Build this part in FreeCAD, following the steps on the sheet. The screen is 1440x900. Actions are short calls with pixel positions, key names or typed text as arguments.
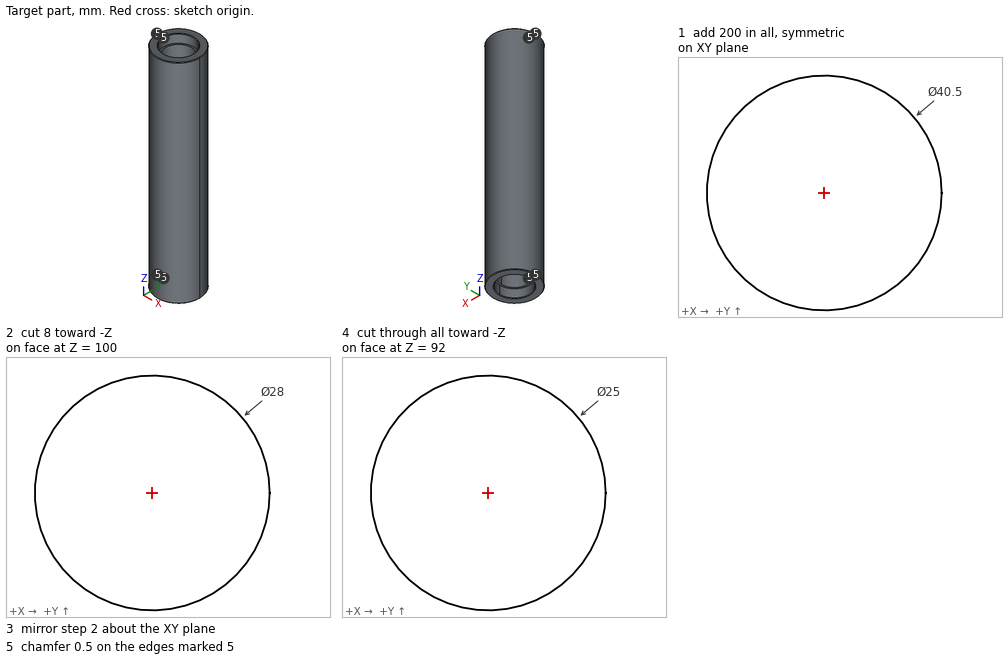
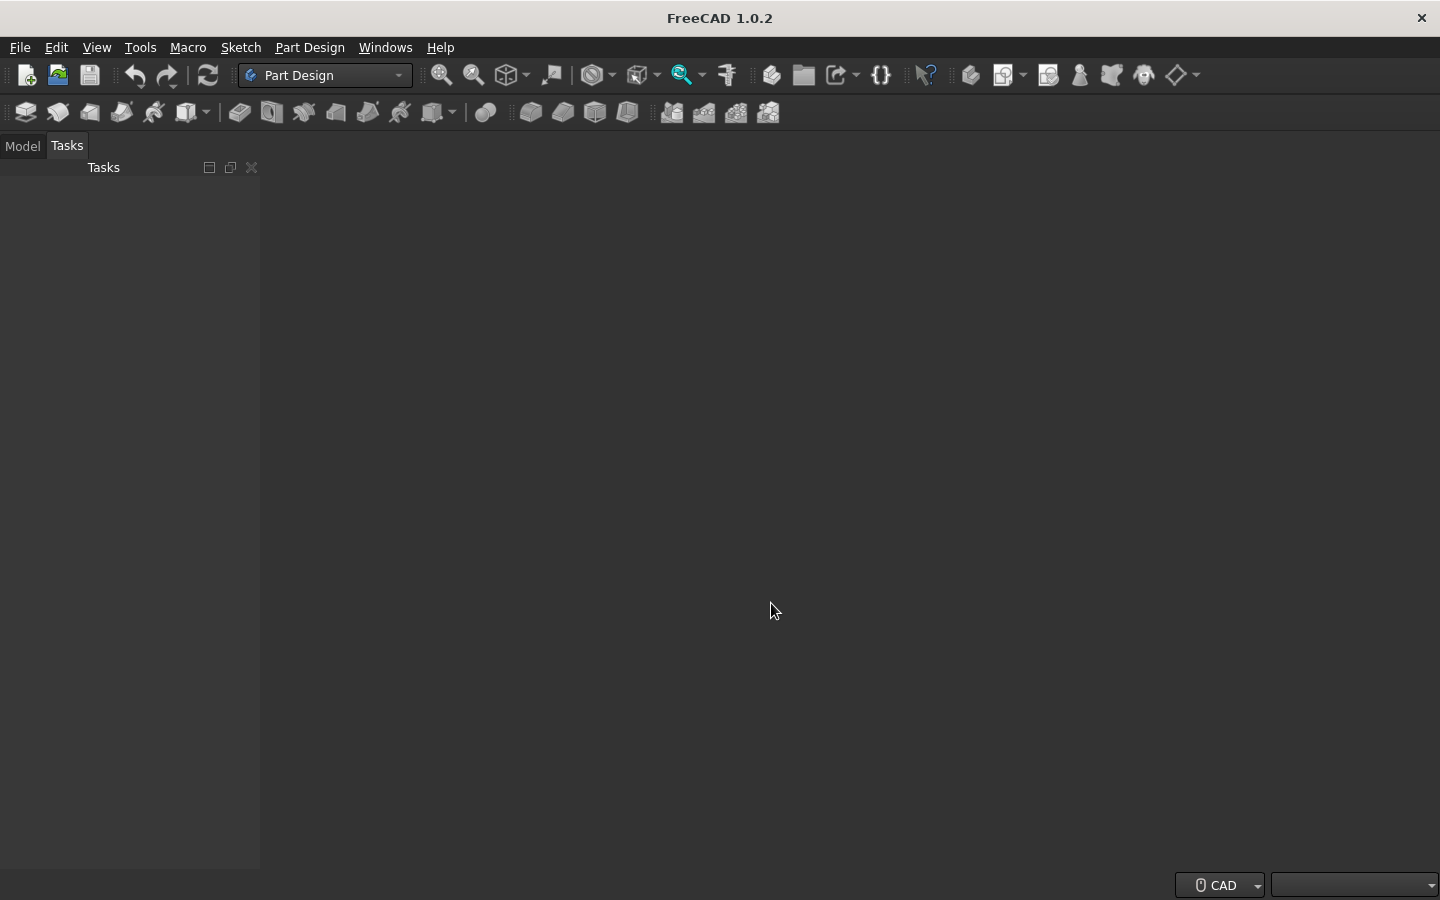
click(26, 76)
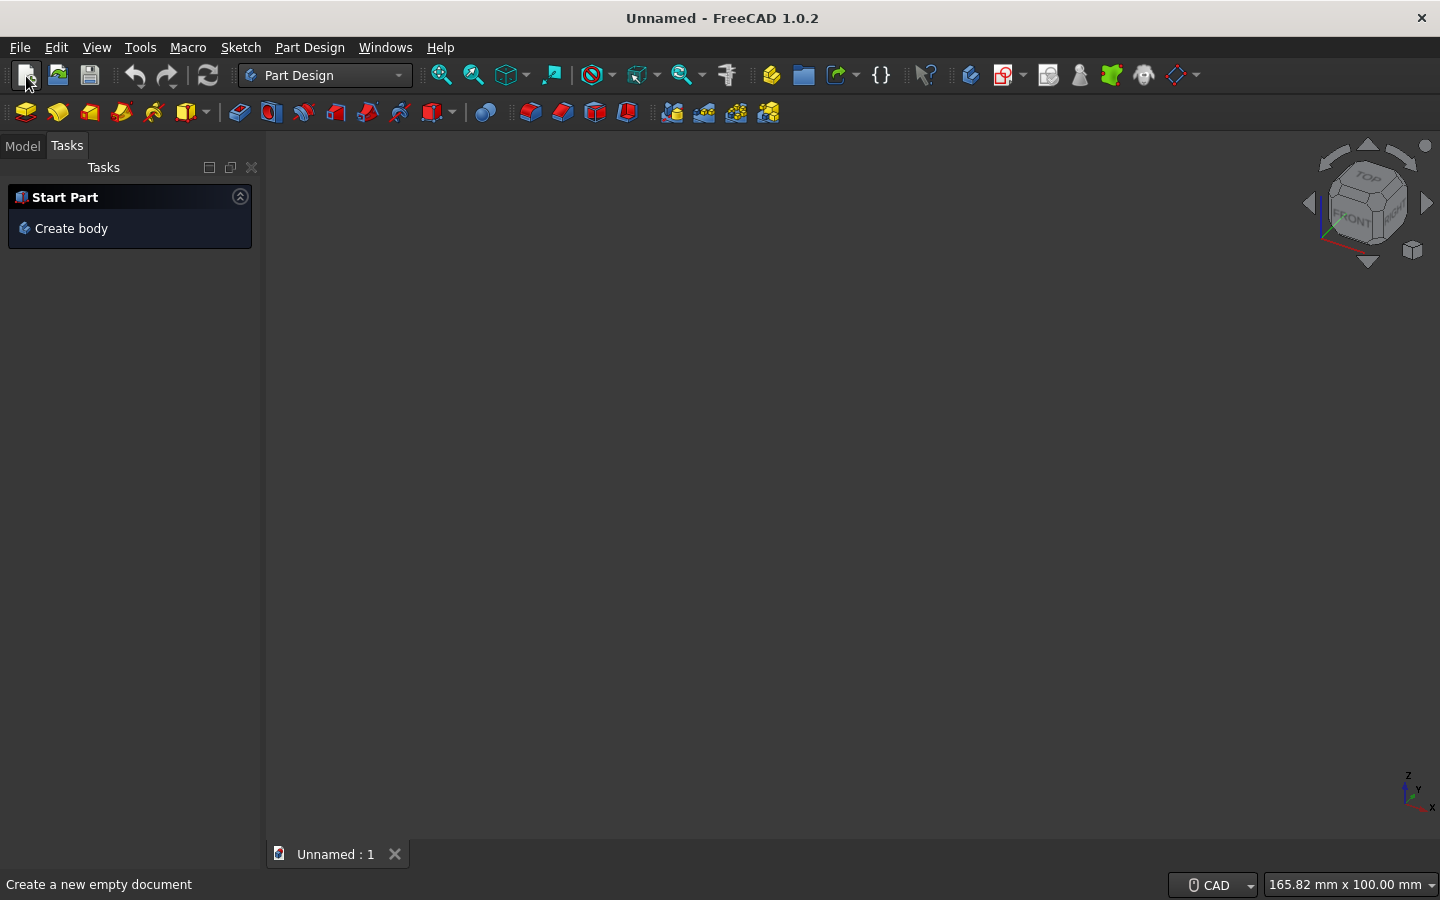
click(1004, 76)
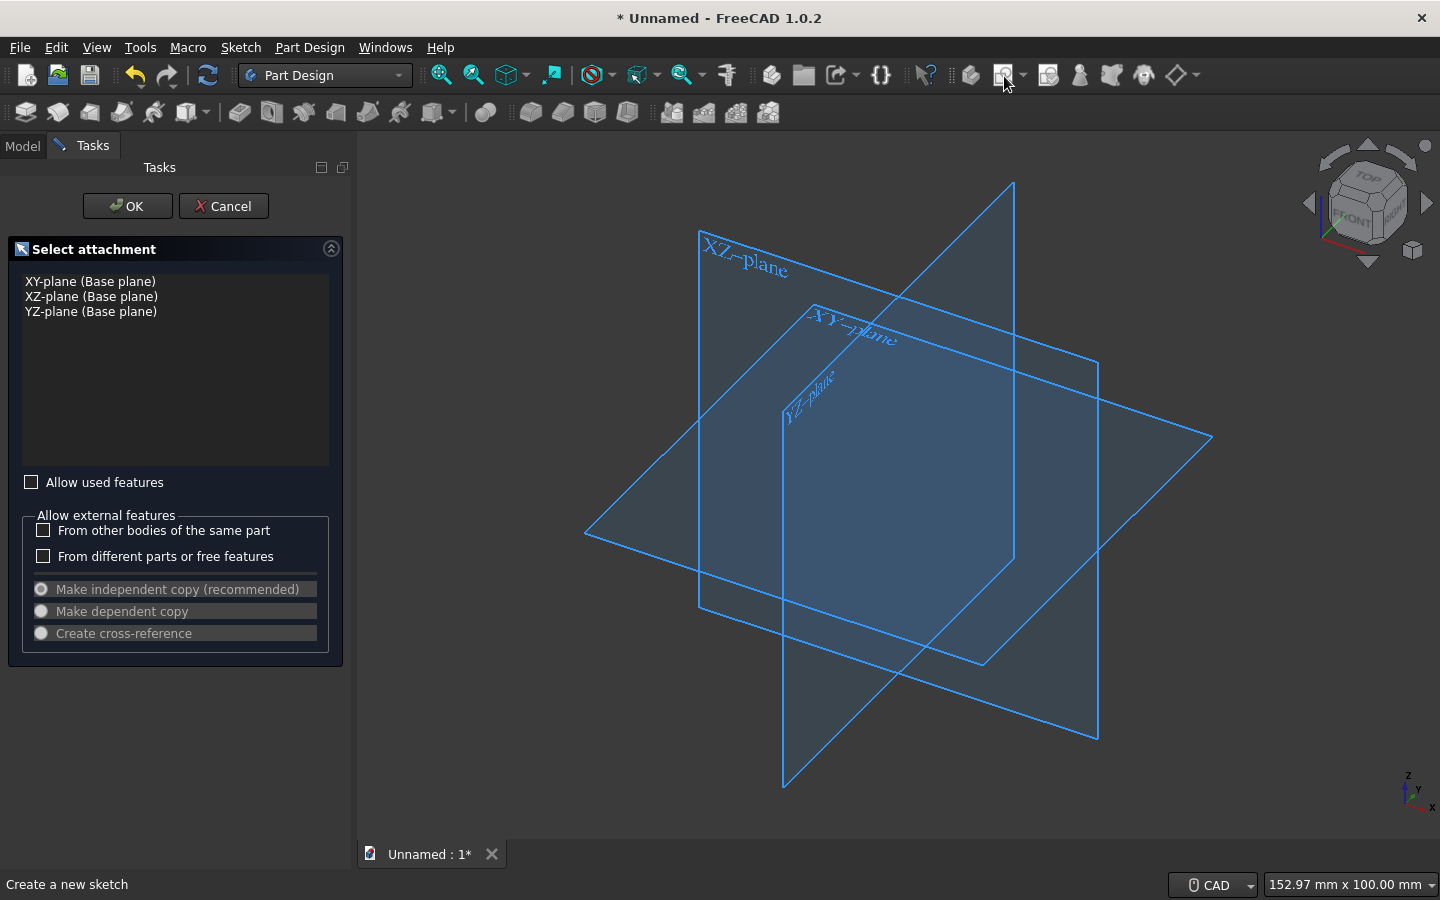
click(82, 282)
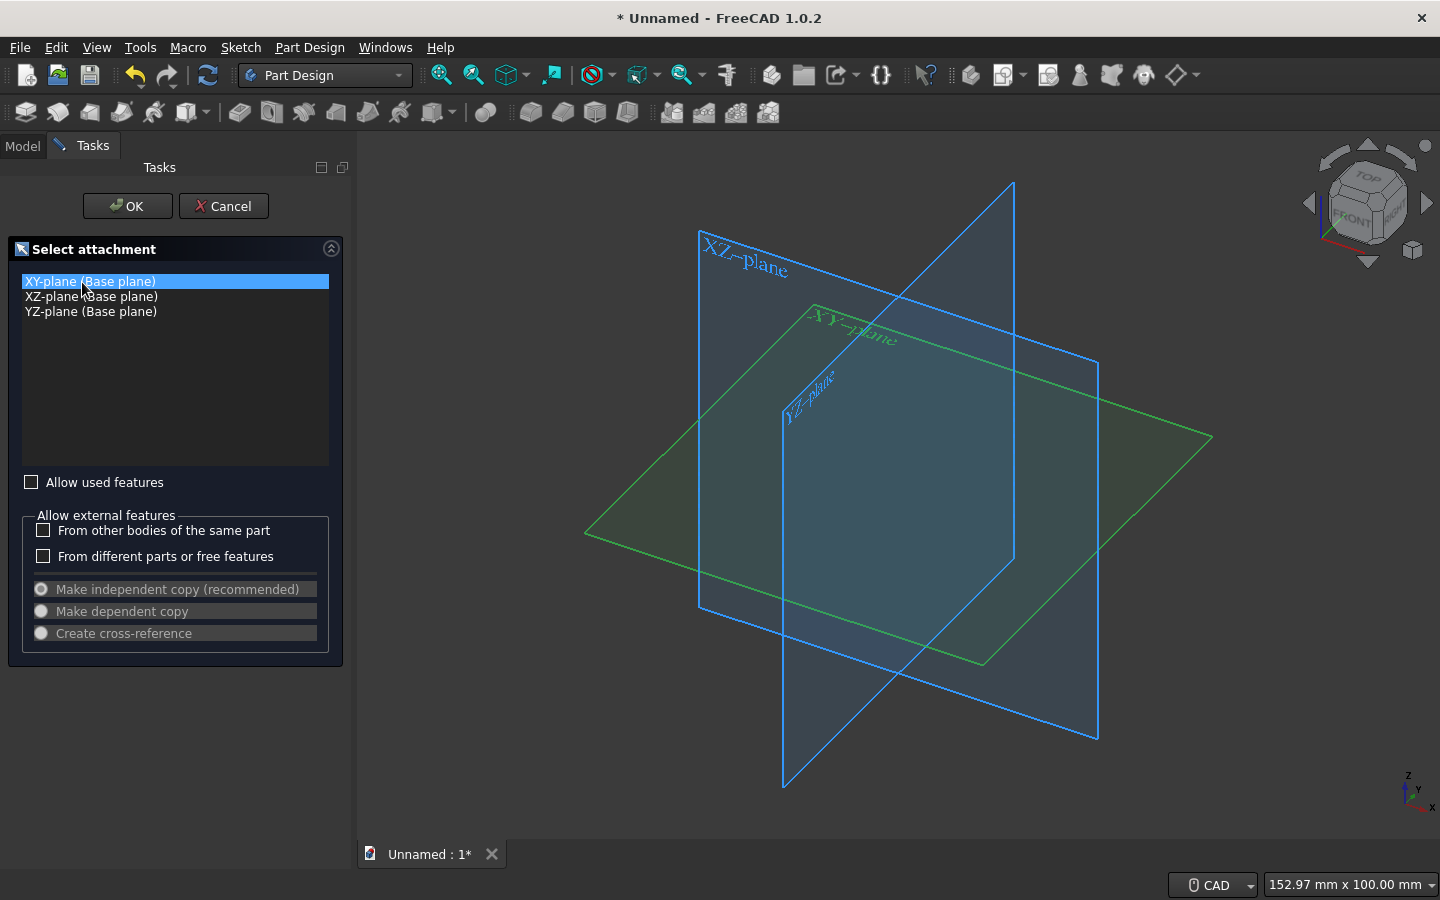
click(128, 206)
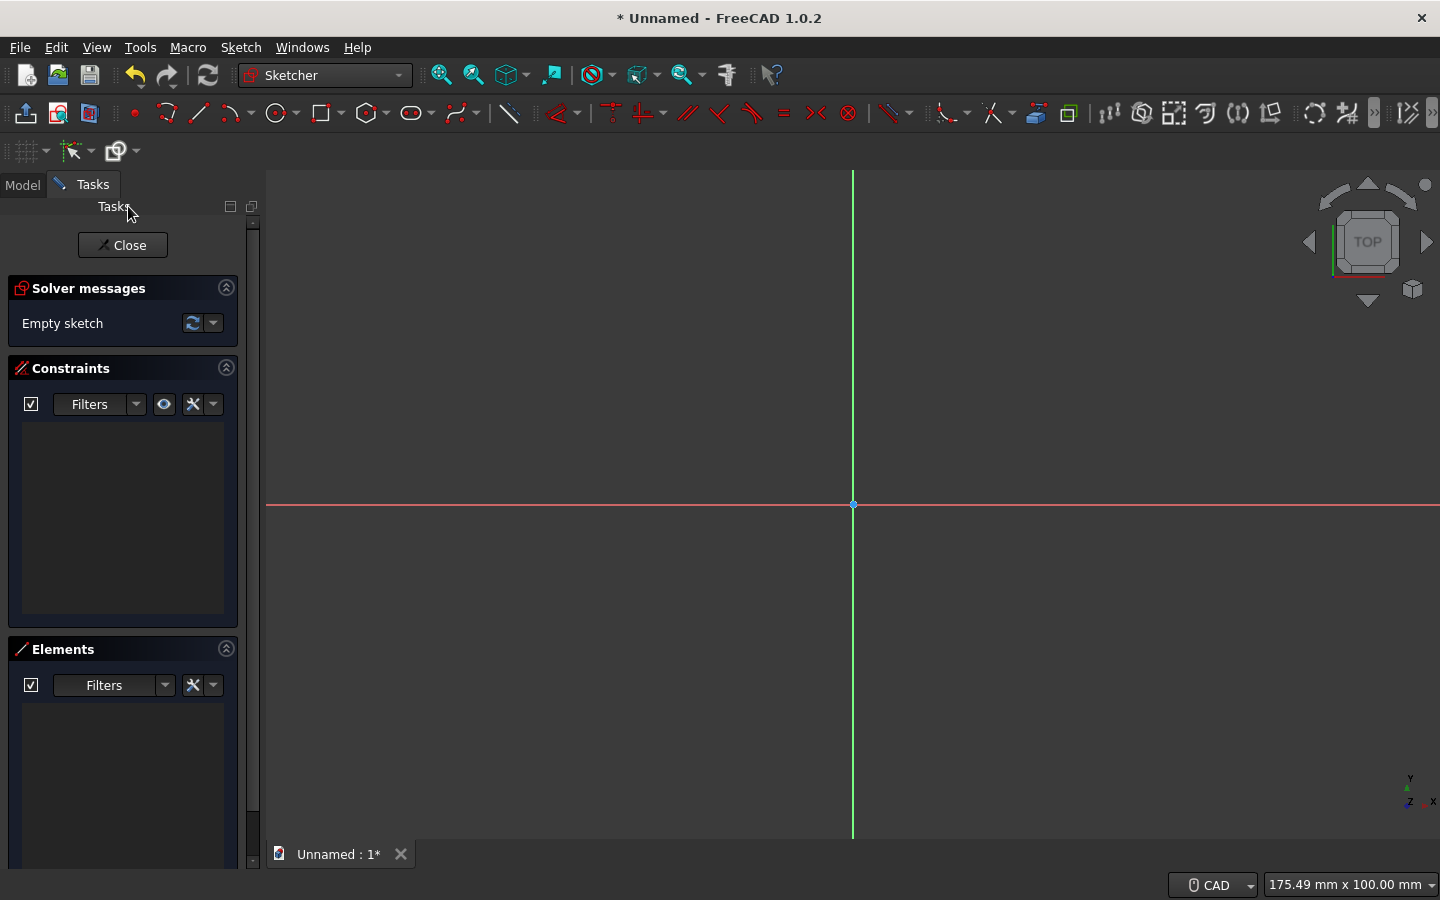
scroll(992, 504, up, 2)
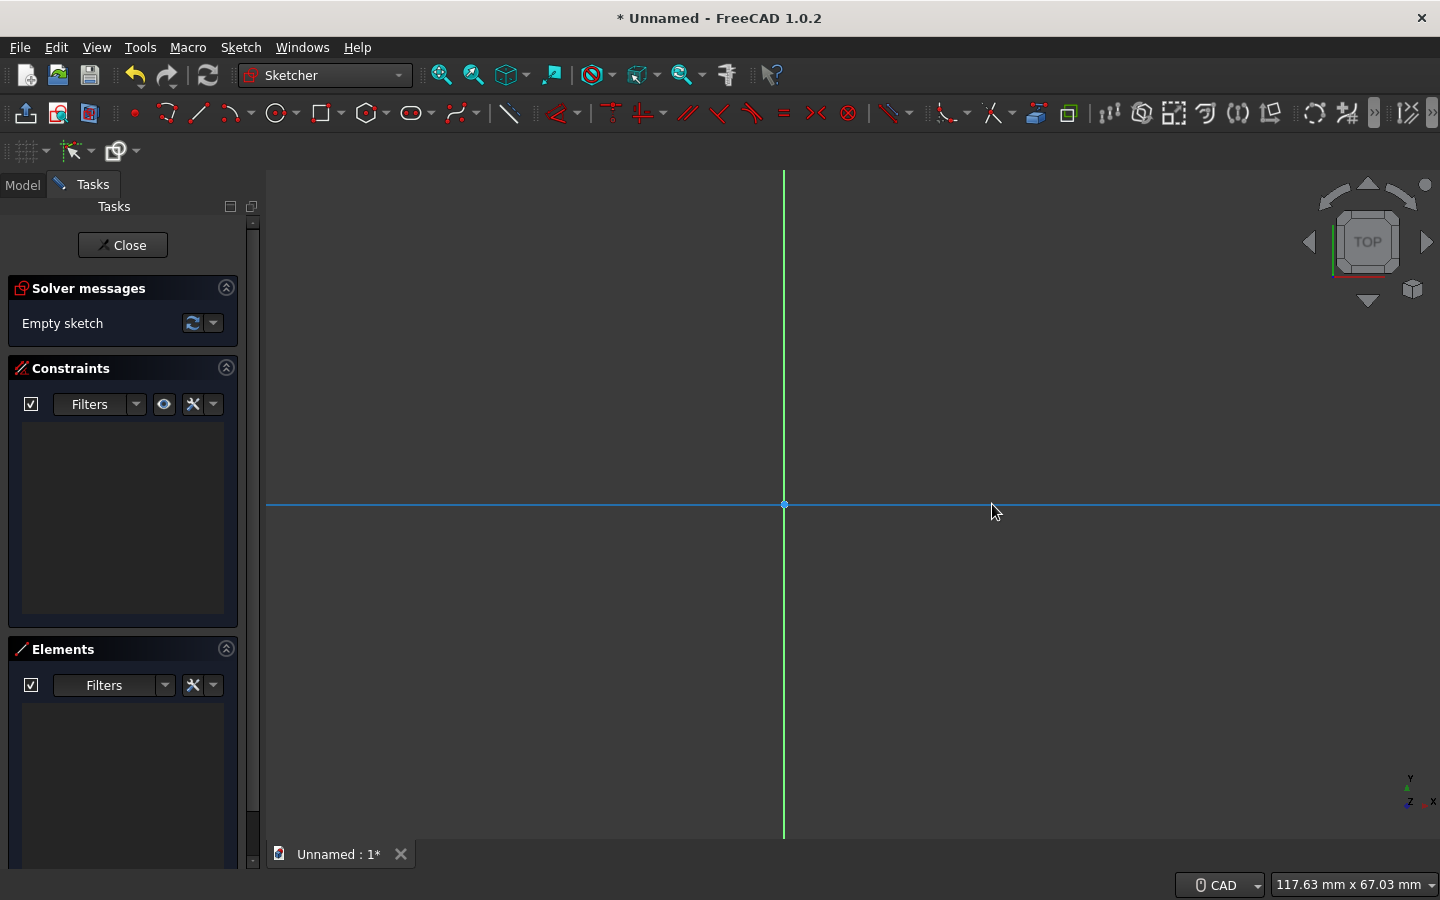
click(276, 114)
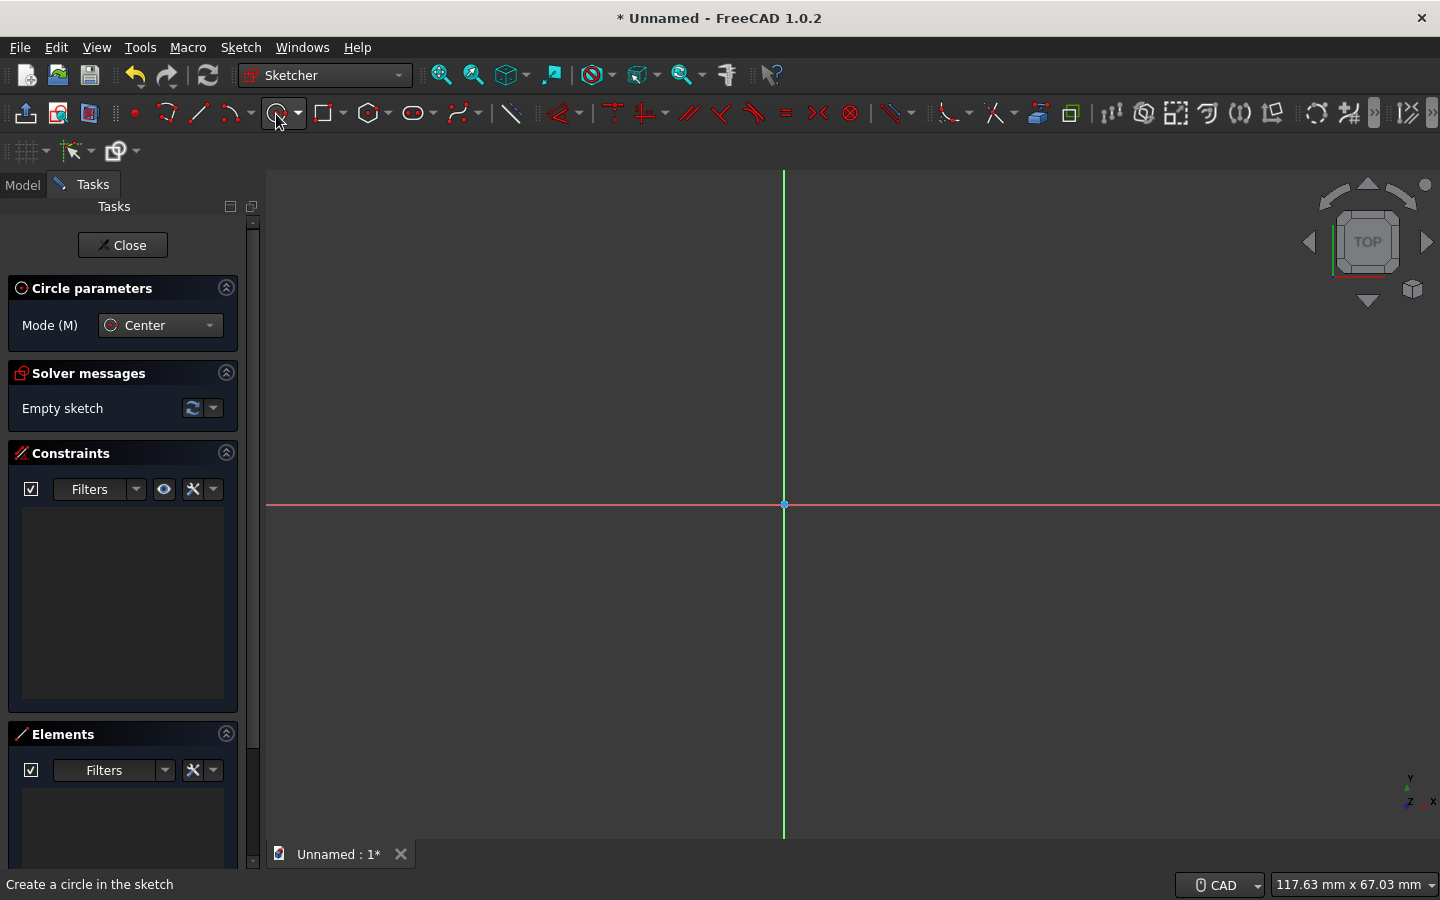
click(784, 504)
move(927, 362)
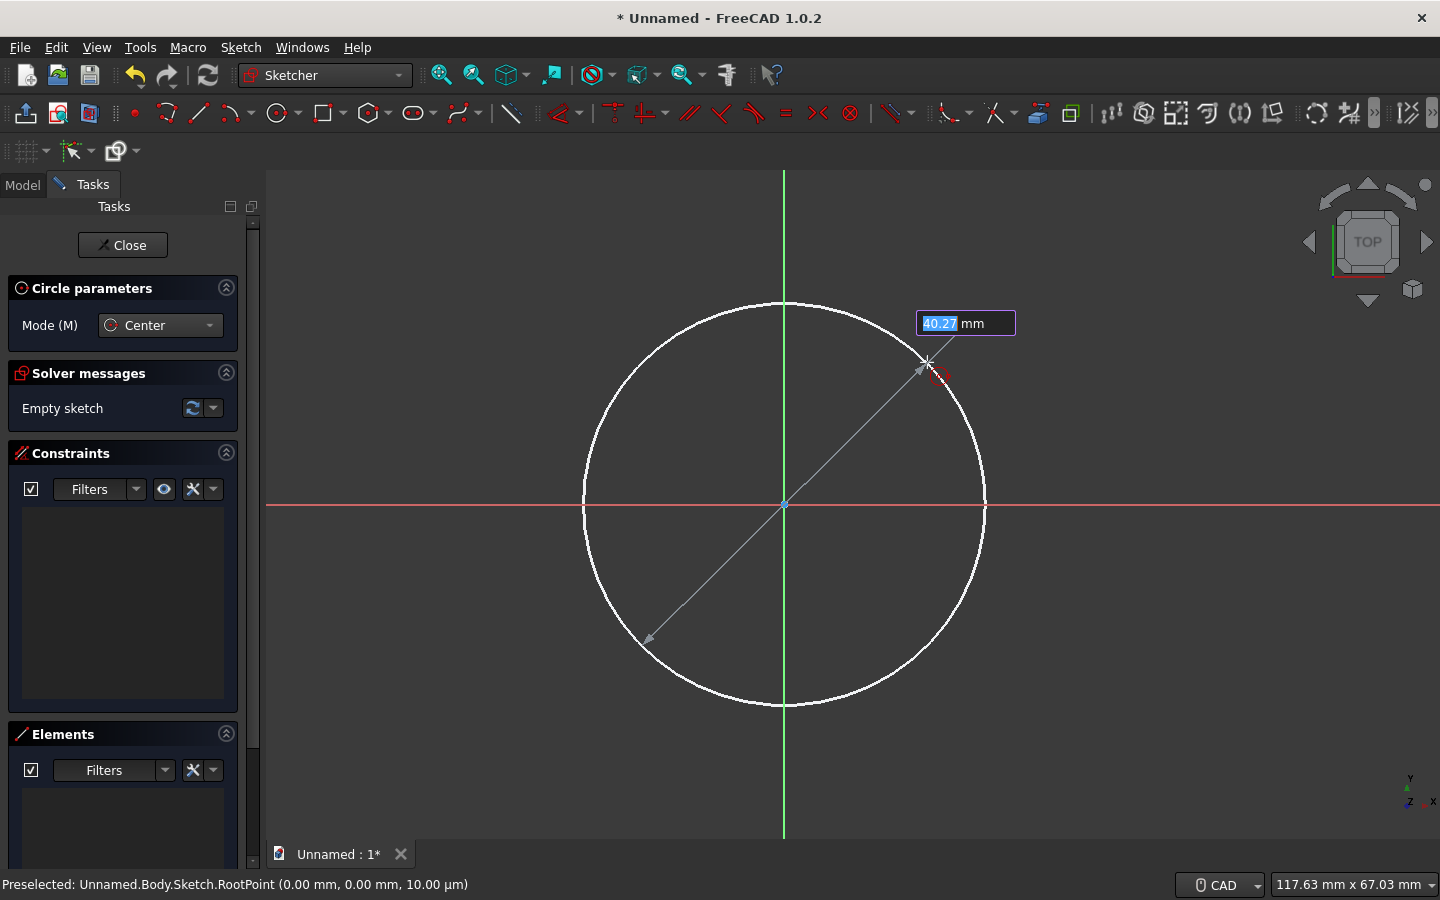
text(40.5)
key(Return)
key(Escape)